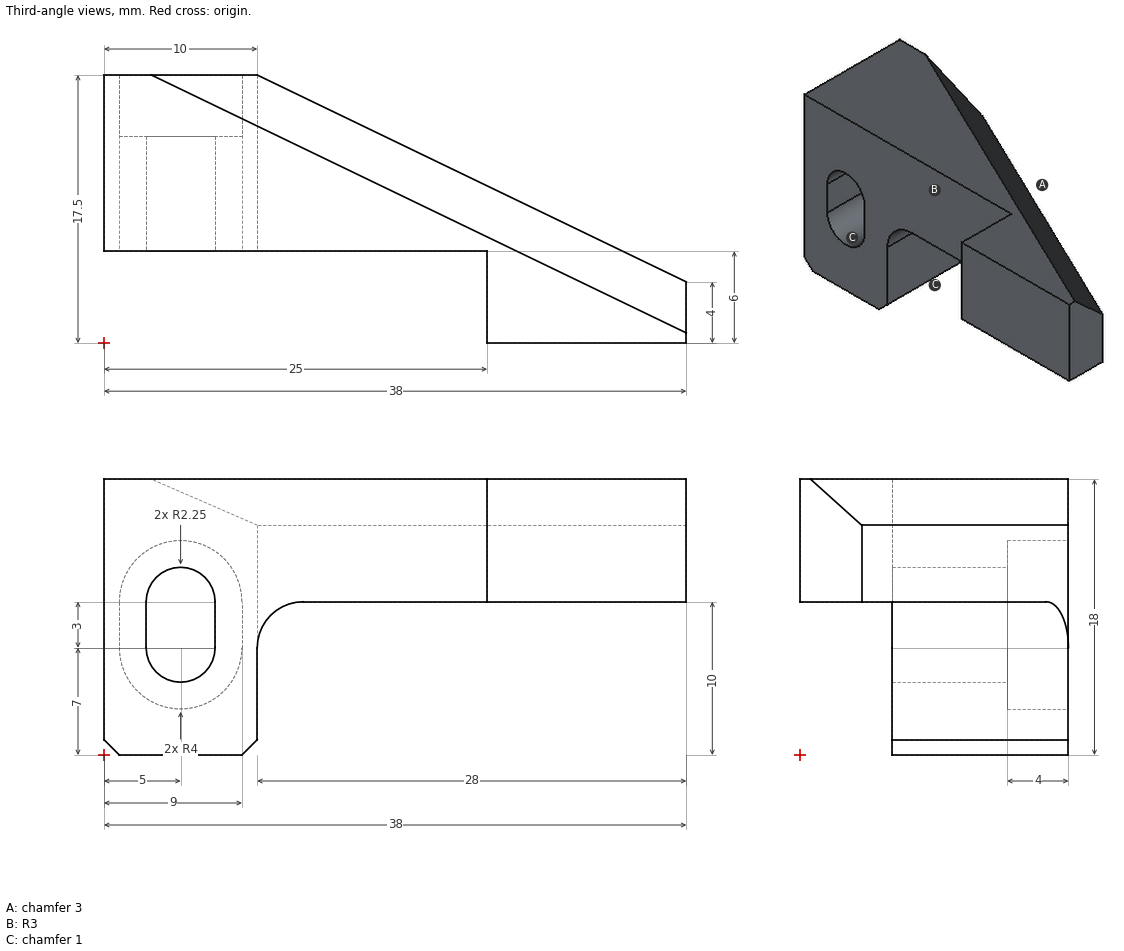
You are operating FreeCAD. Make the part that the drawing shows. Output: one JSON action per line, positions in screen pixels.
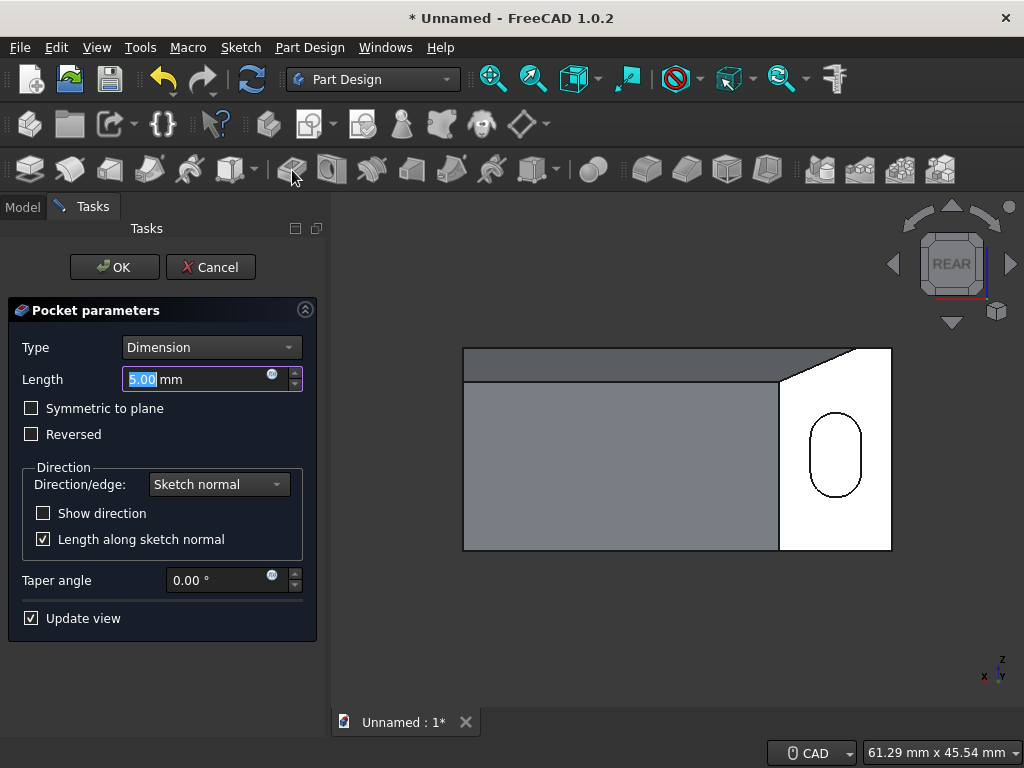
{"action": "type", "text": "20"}
{"action": "key", "text": "Tab"}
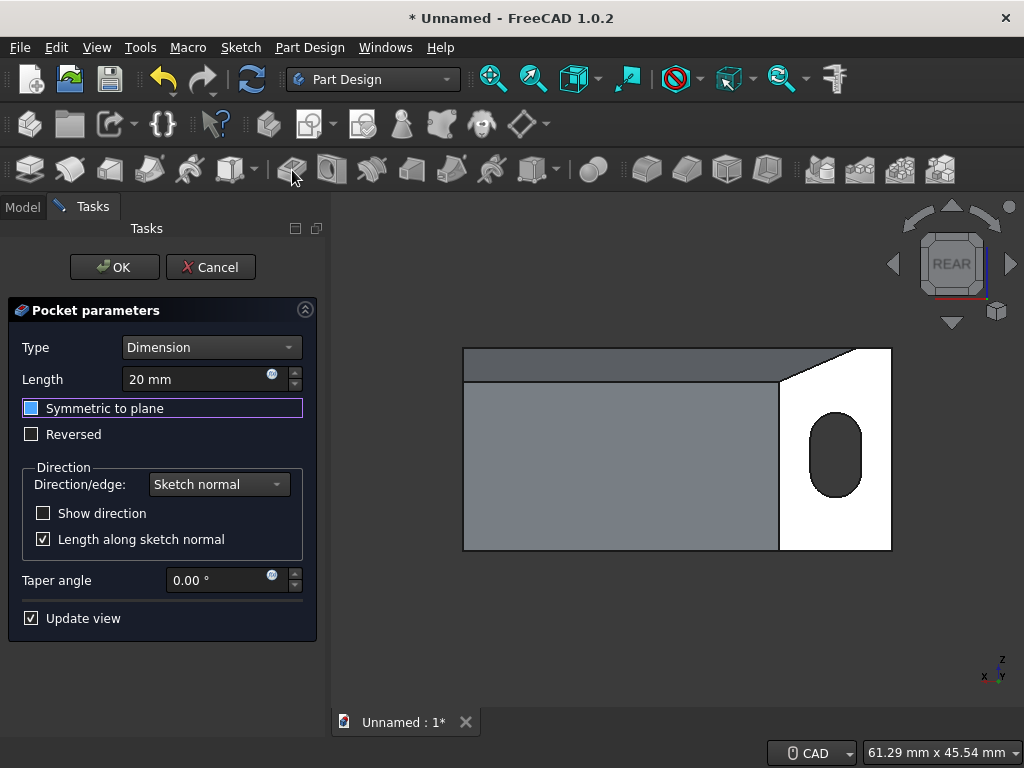
{"action": "left_click", "coordinate": [115, 267]}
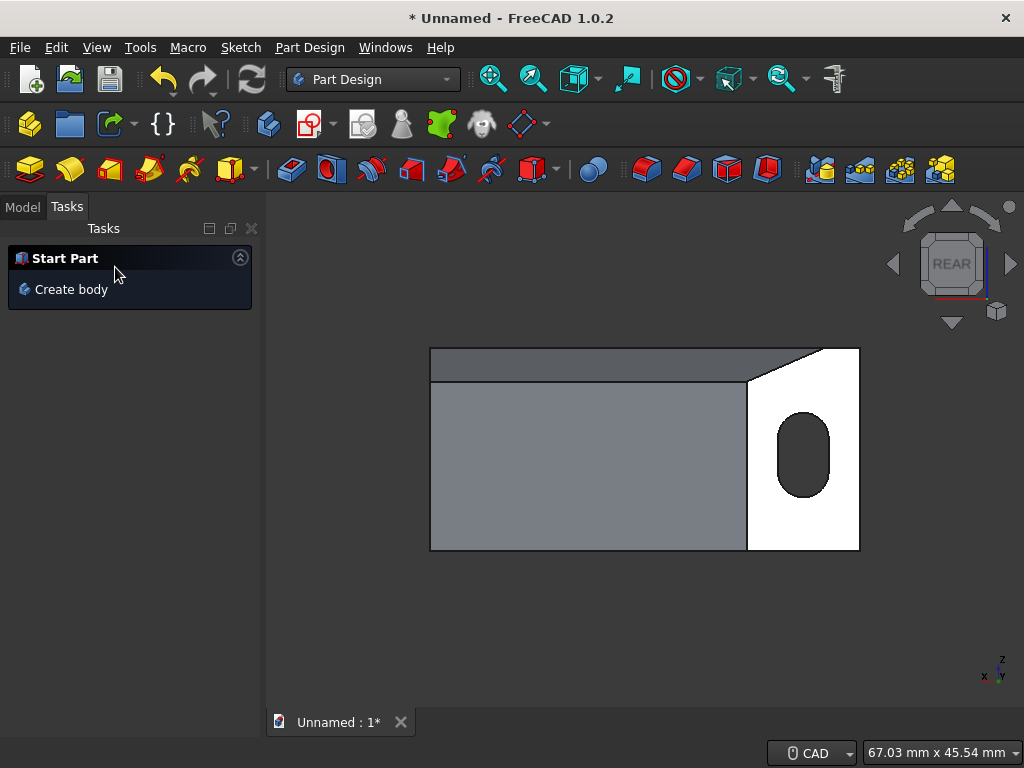
{"action": "left_click", "coordinate": [836, 390]}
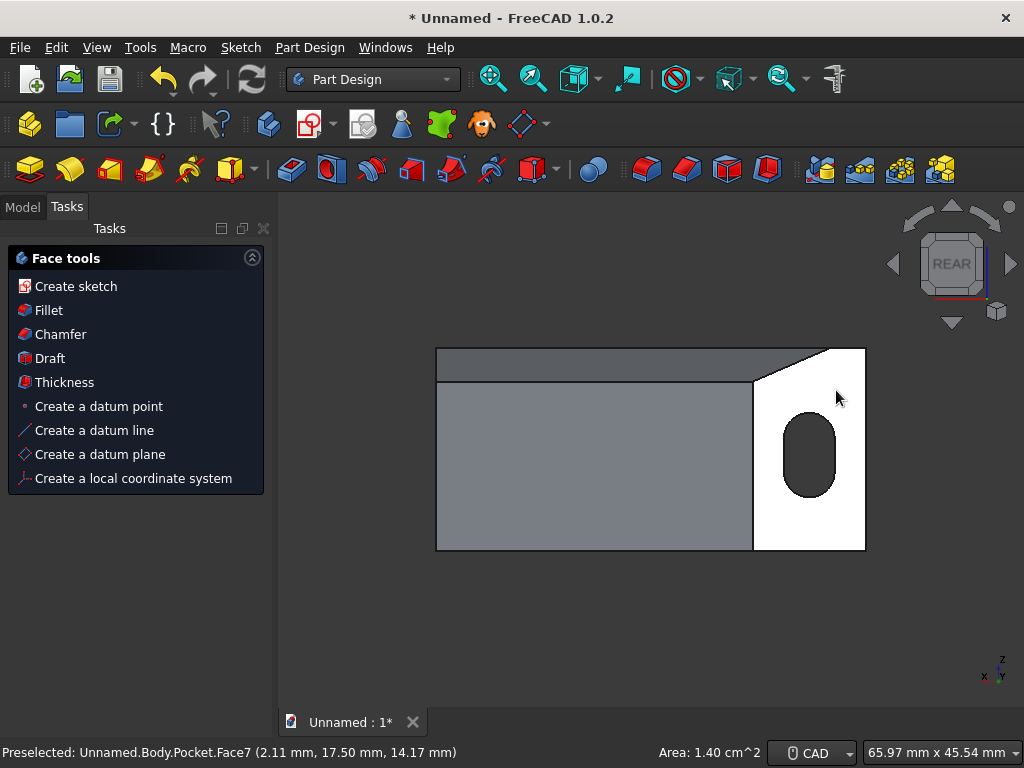
{"action": "left_click", "coordinate": [310, 124]}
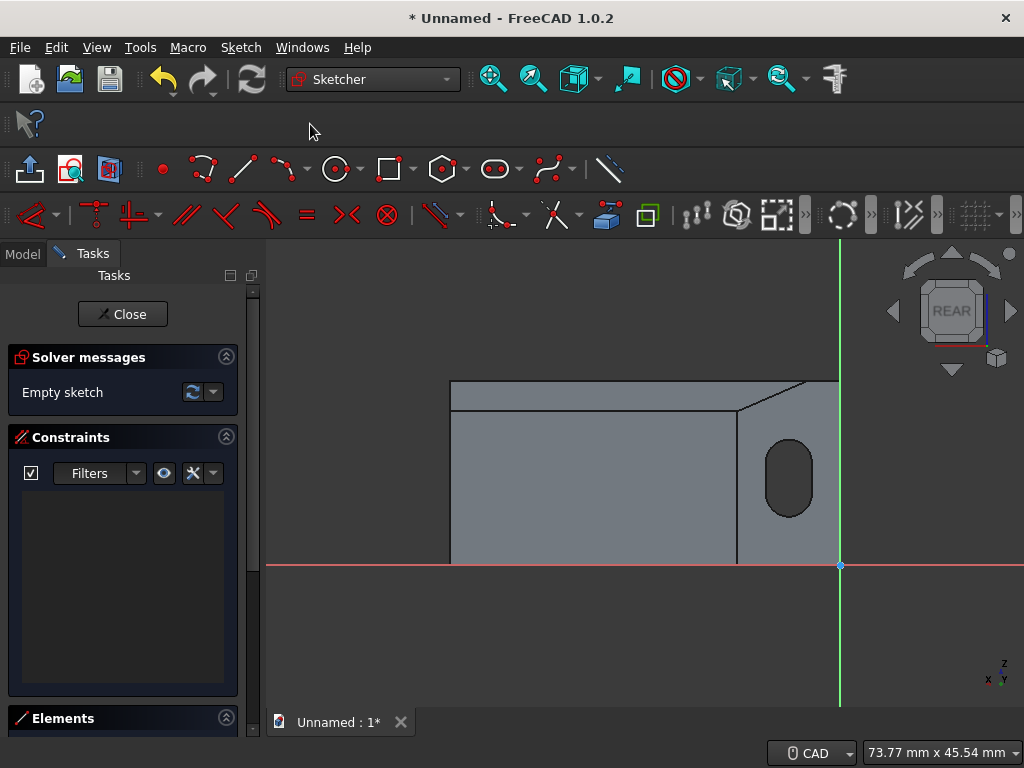
{"action": "scroll", "coordinate": [859, 510], "scroll_direction": "up", "scroll_amount": 4}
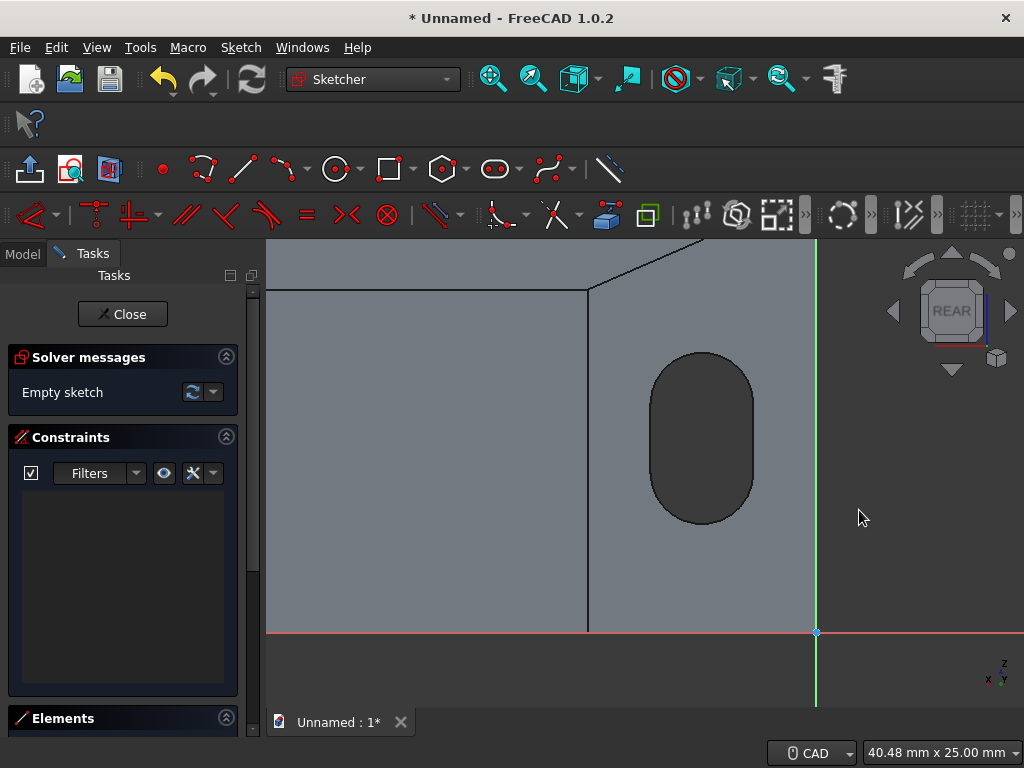
{"action": "key", "text": "g s"}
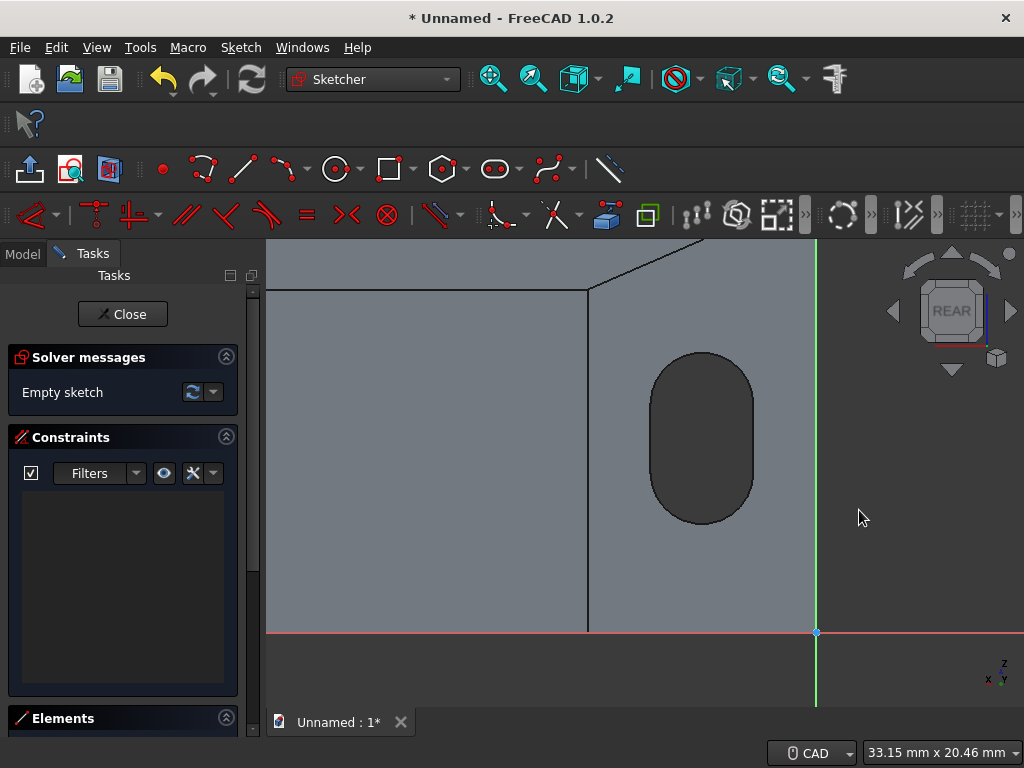
{"action": "left_click", "coordinate": [702, 473]}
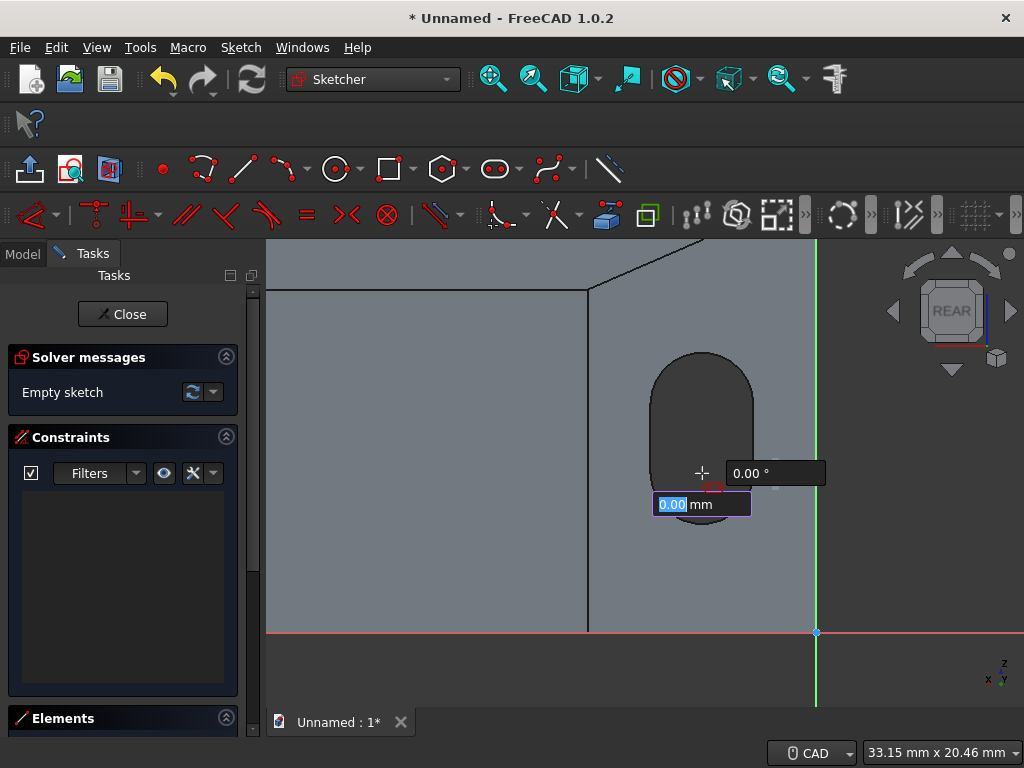
{"action": "left_click", "coordinate": [702, 404]}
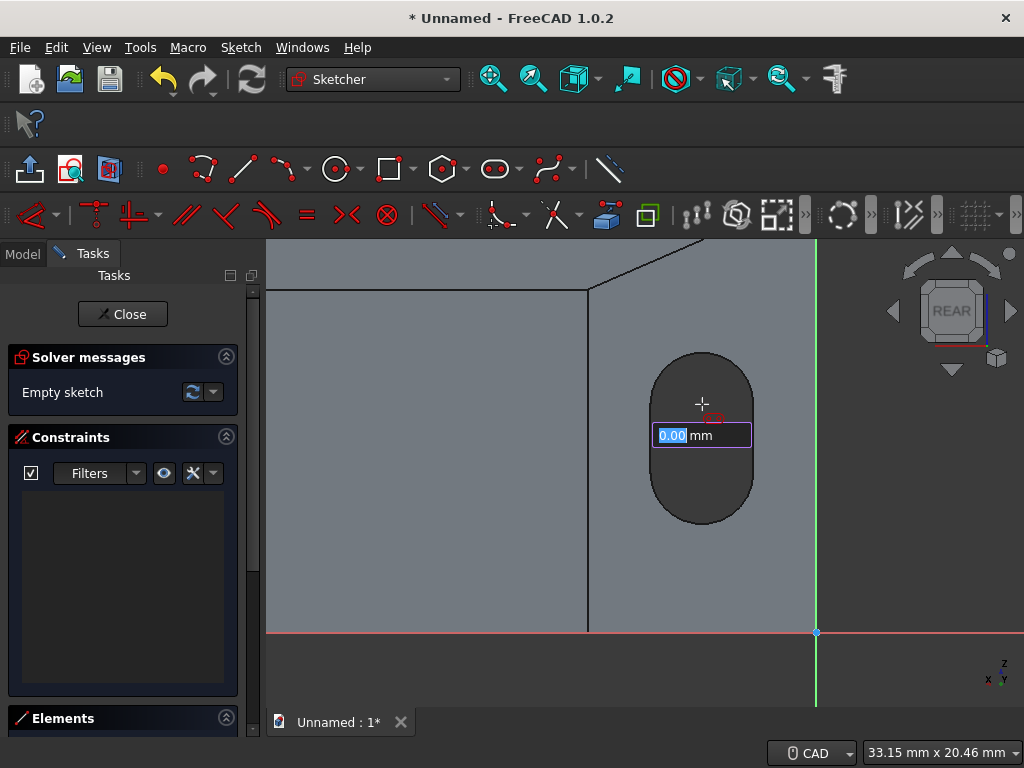
{"action": "left_click", "coordinate": [610, 438]}
{"action": "key", "text": "Escape"}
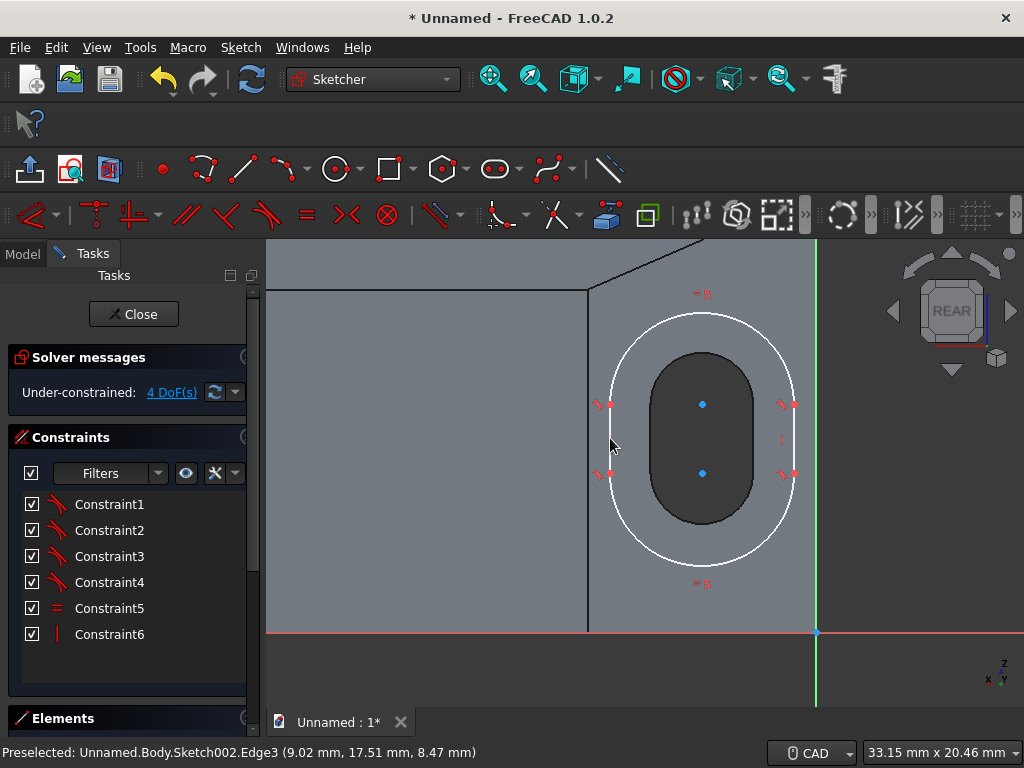
{"action": "key", "text": "d"}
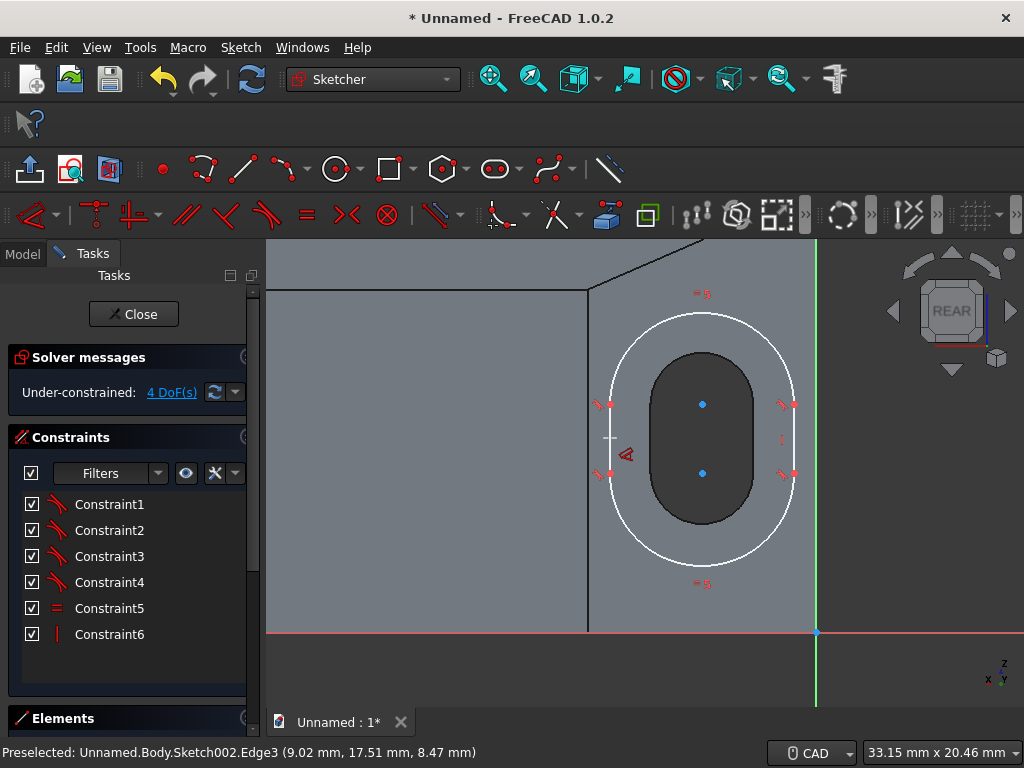
{"action": "left_click", "coordinate": [648, 548]}
{"action": "left_click", "coordinate": [629, 574]}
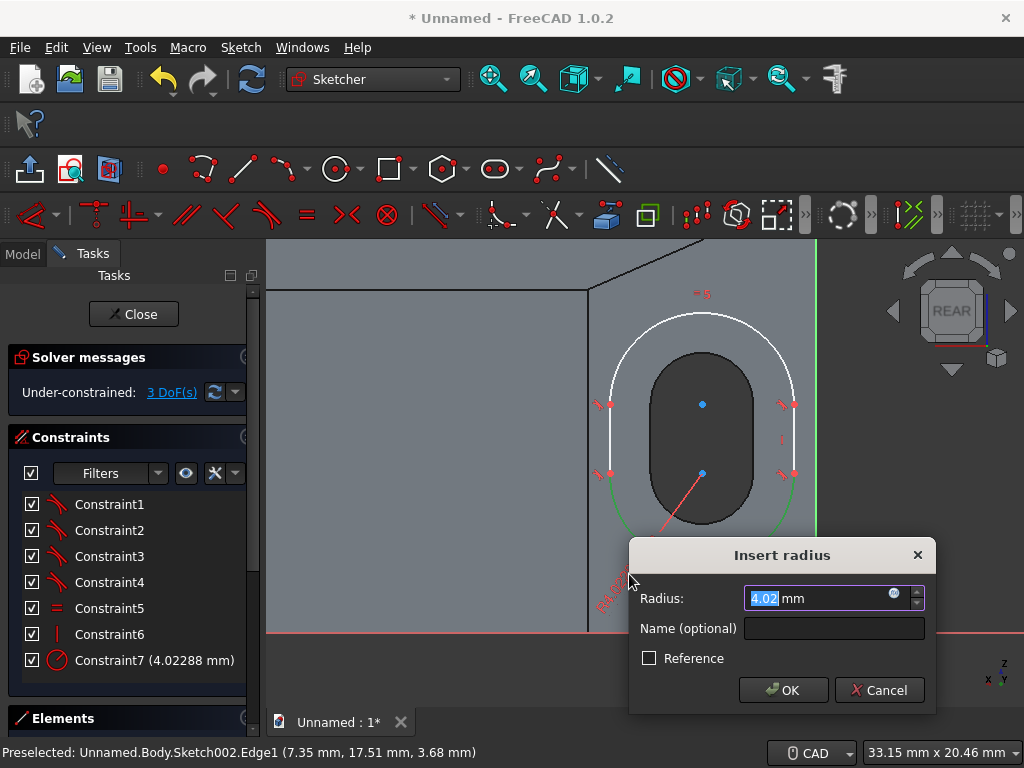
{"action": "type", "text": "4"}
{"action": "key", "text": "Return"}